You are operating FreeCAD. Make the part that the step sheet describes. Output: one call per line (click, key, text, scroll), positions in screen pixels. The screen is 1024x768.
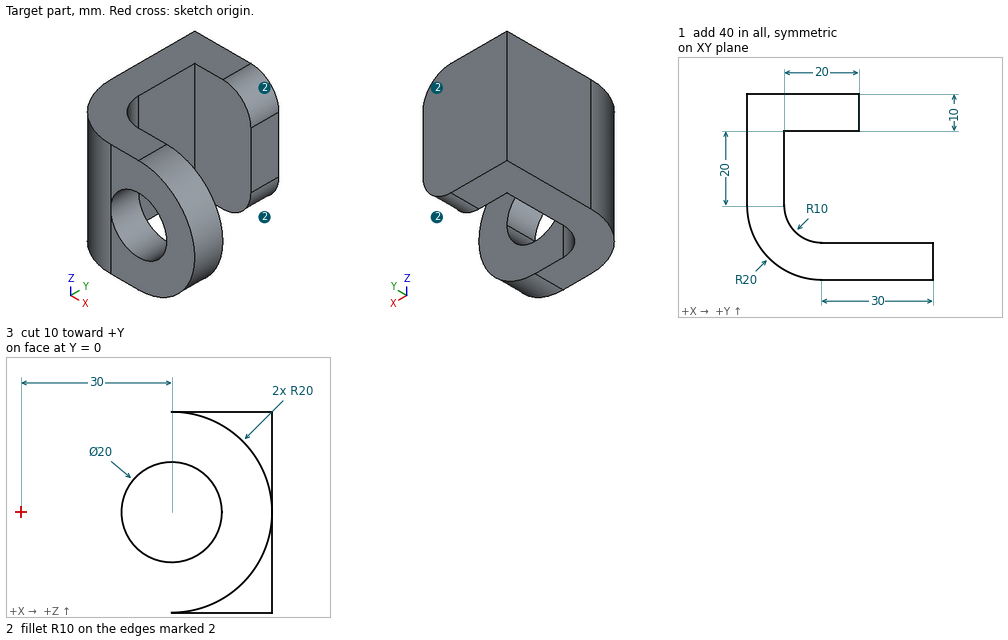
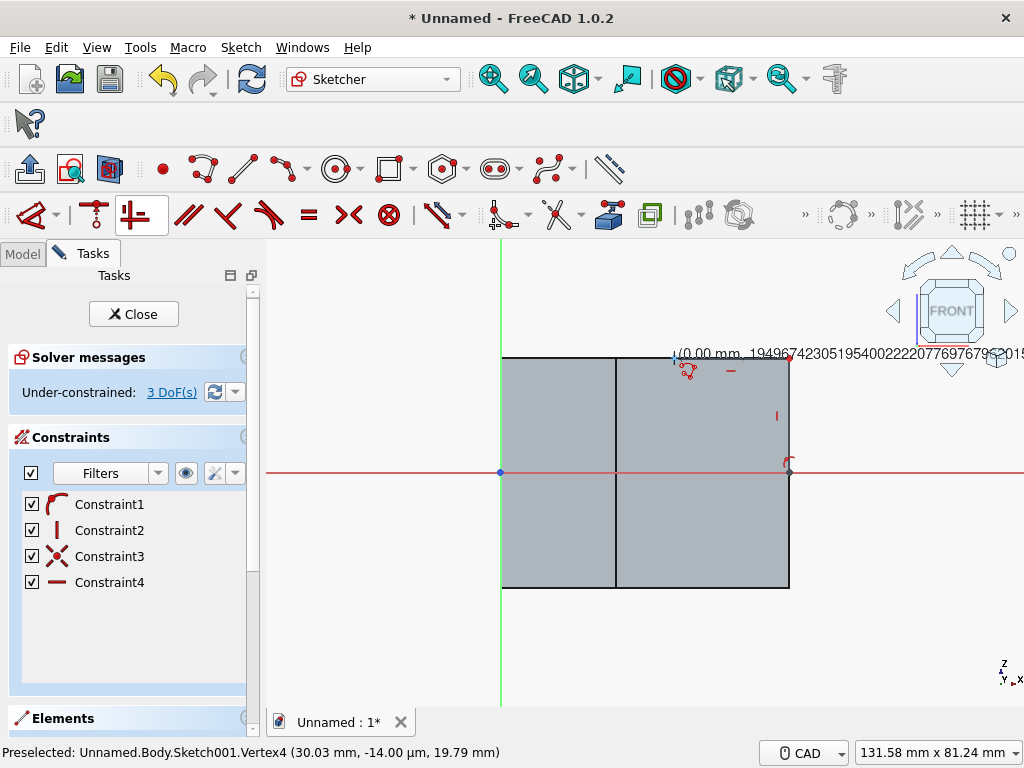
click(284, 170)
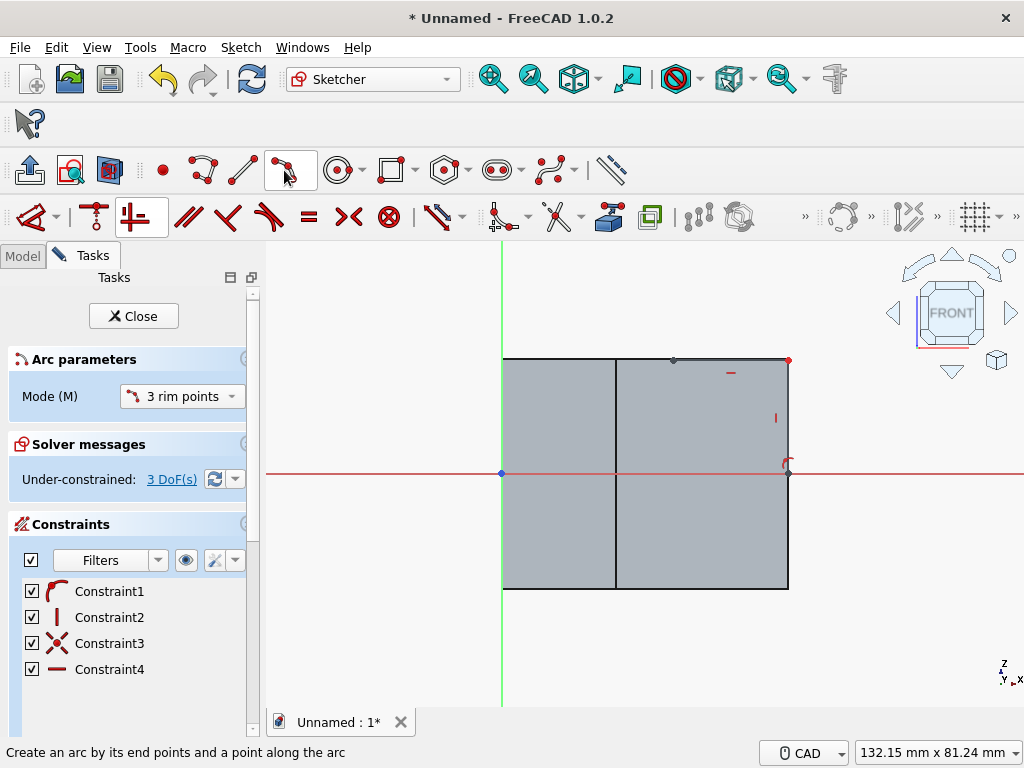
click(674, 360)
click(788, 474)
click(755, 393)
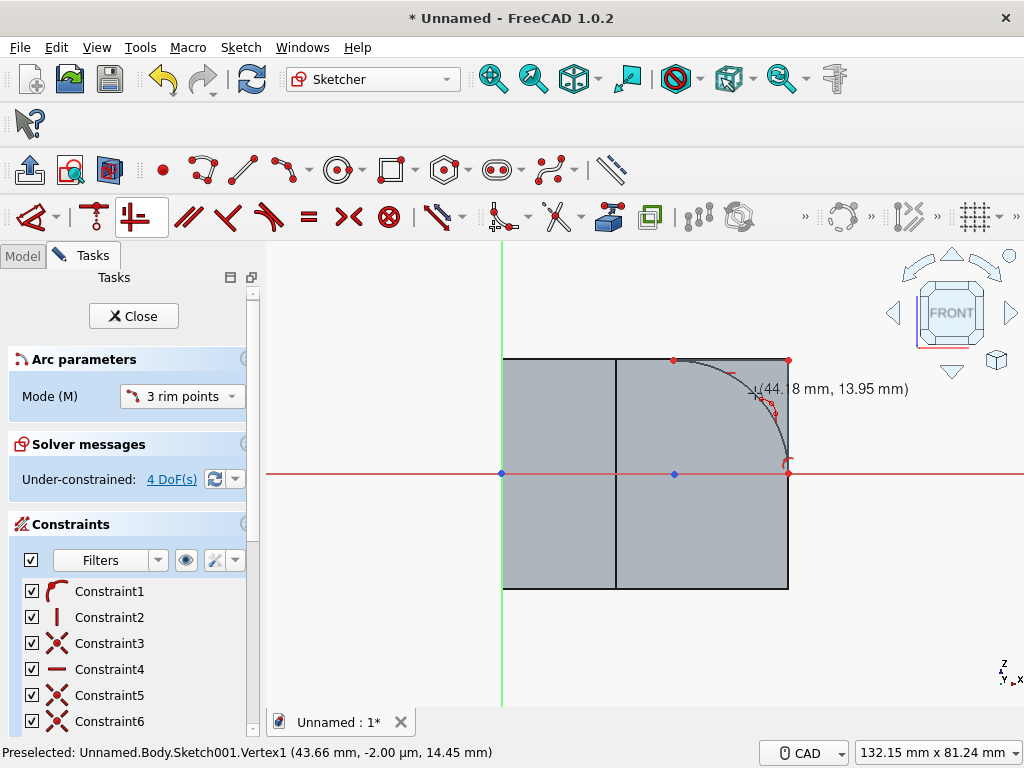
key(g)
key(m)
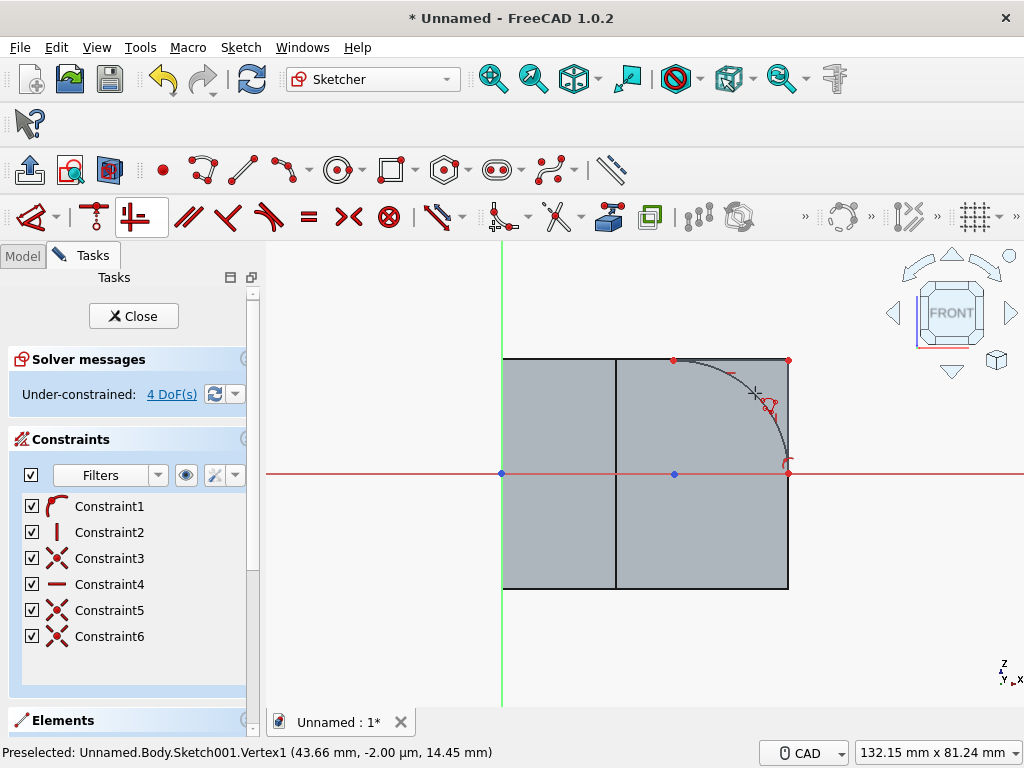
click(674, 589)
click(788, 589)
click(788, 474)
right_click(788, 589)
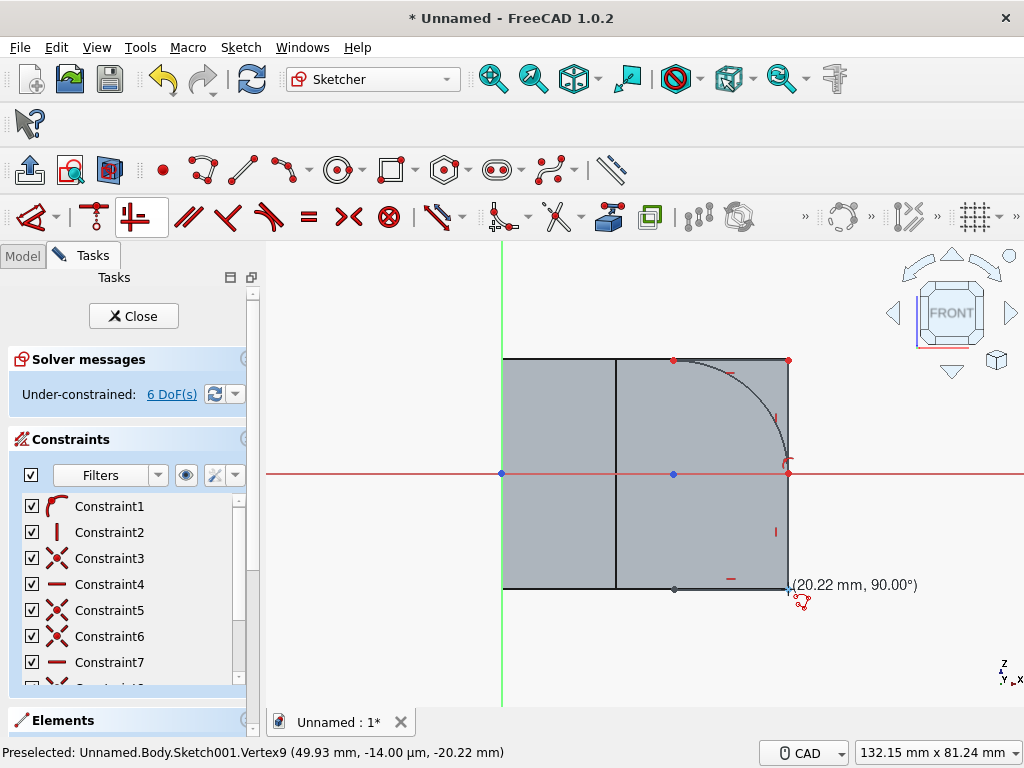
click(284, 170)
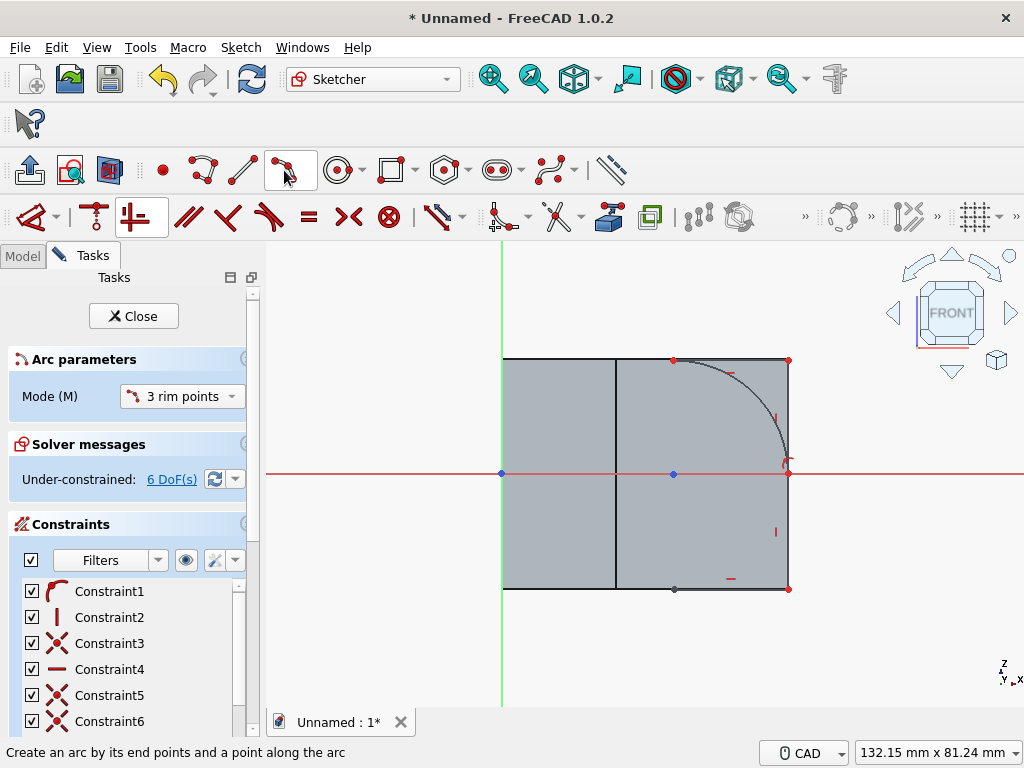
click(788, 474)
click(674, 590)
click(755, 555)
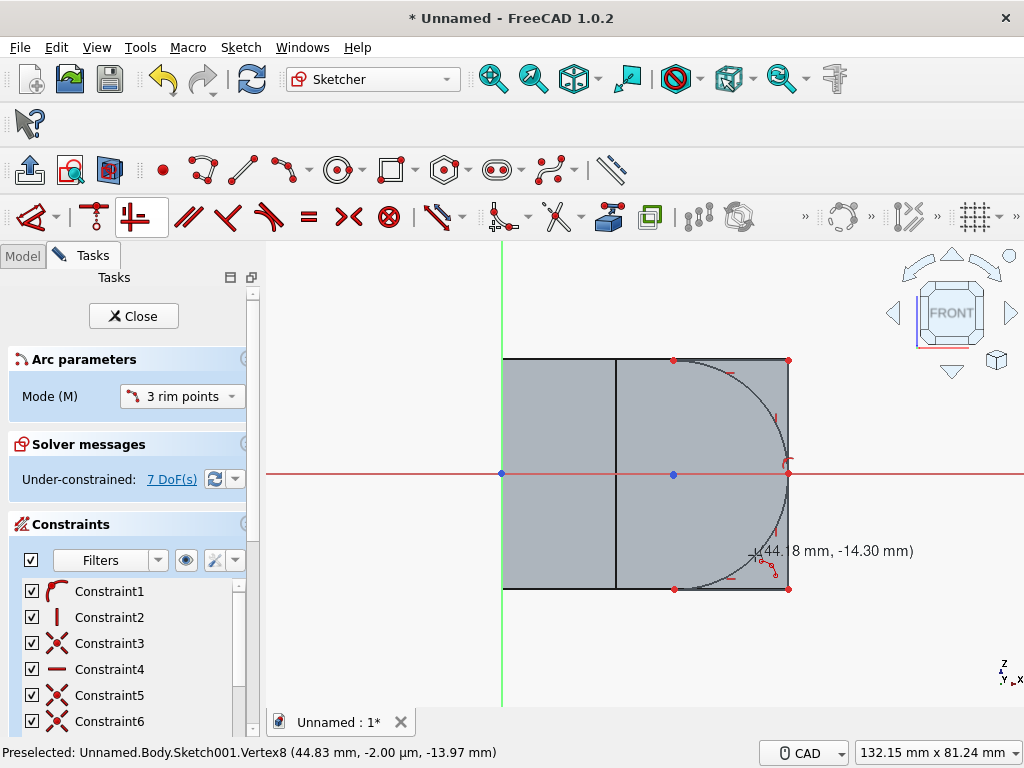
click(338, 170)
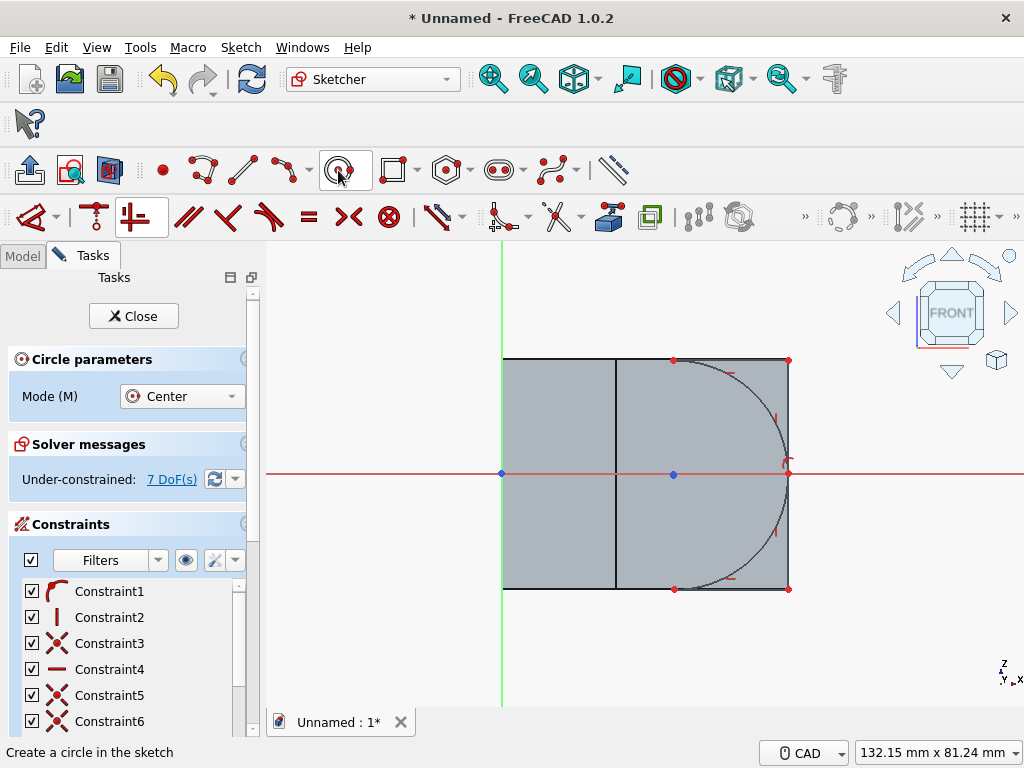
click(674, 474)
move(714, 433)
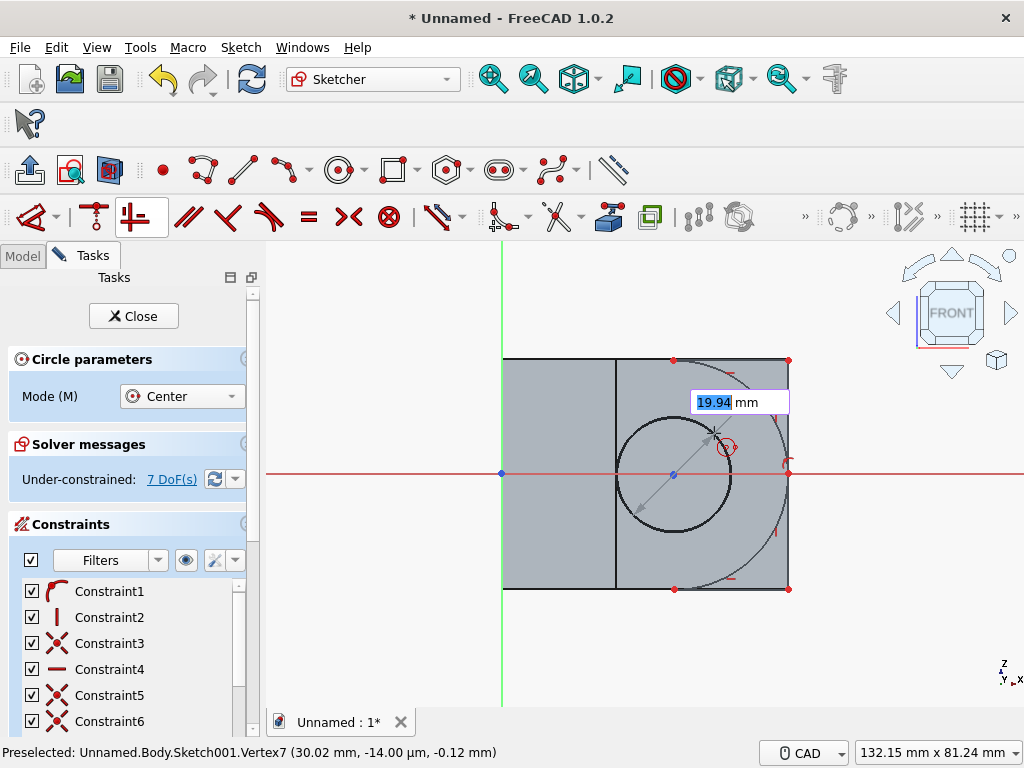
text(20)
key(Return)
key(Escape)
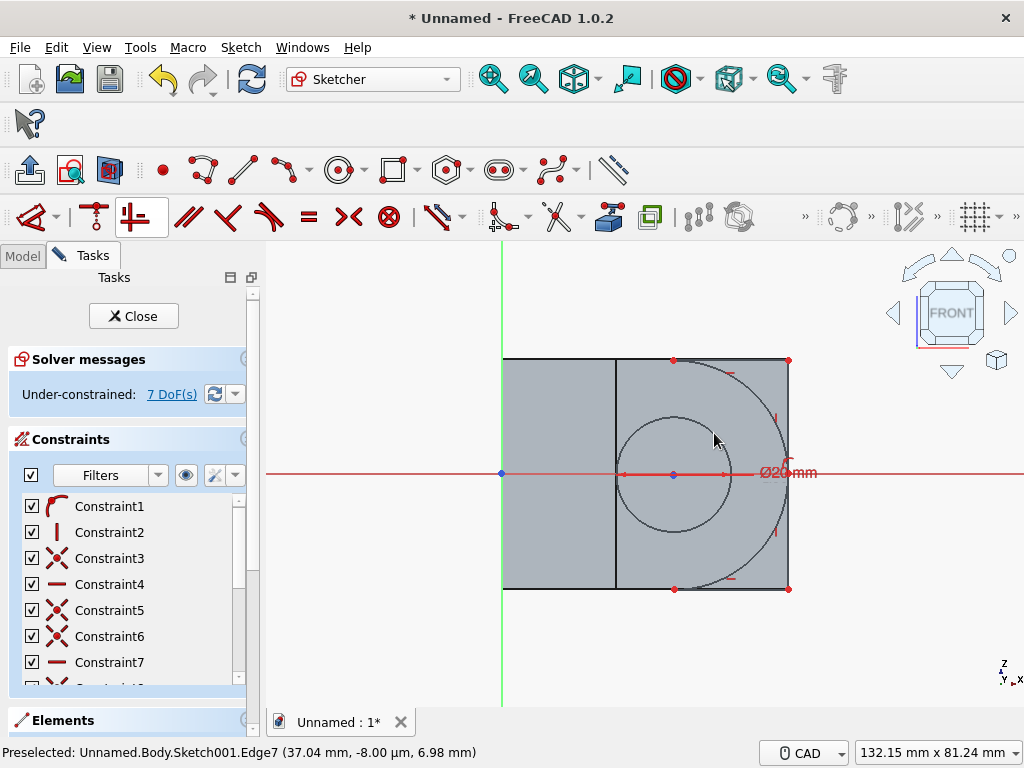
click(788, 395)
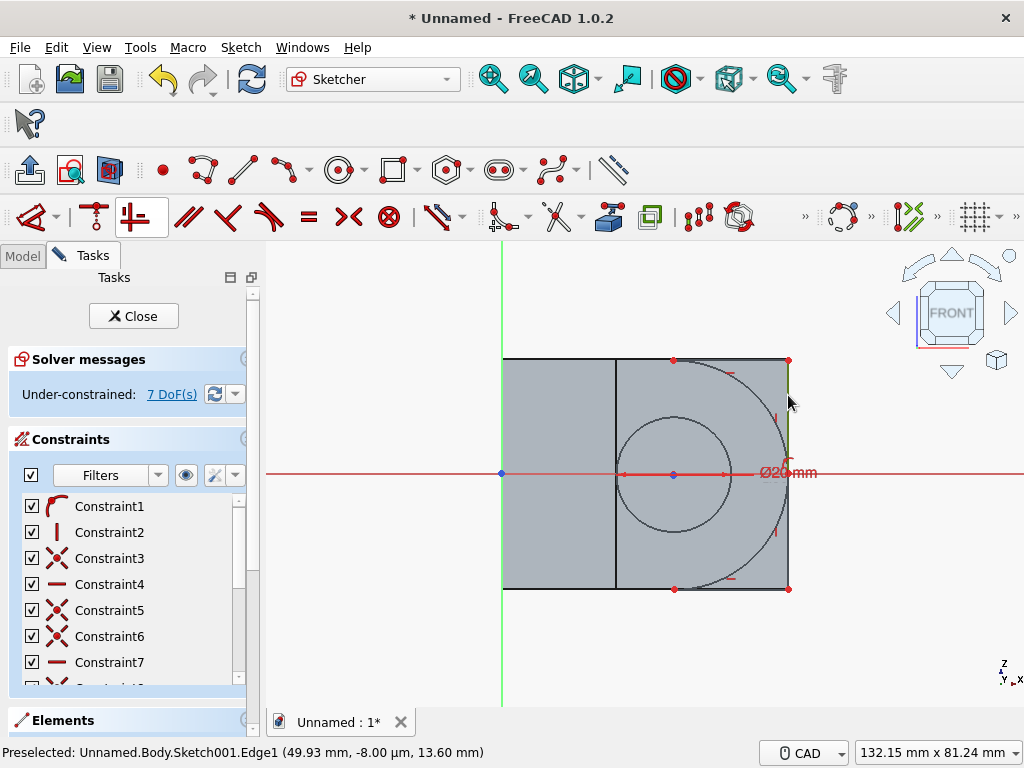
click(754, 394)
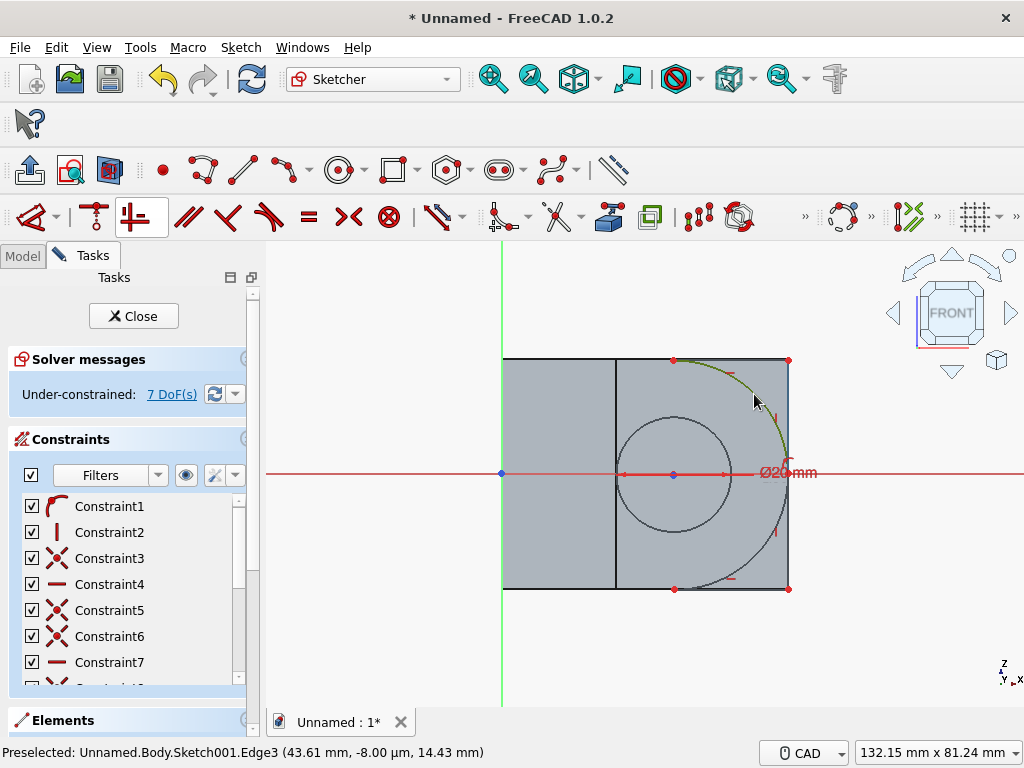
click(270, 218)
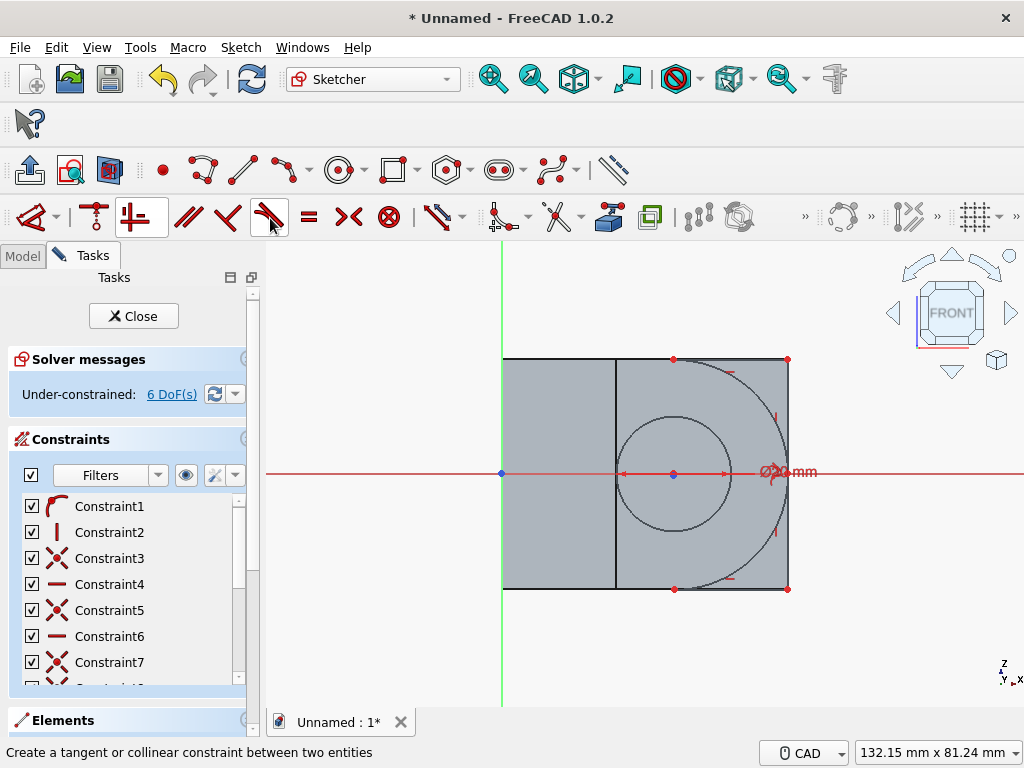
click(788, 394)